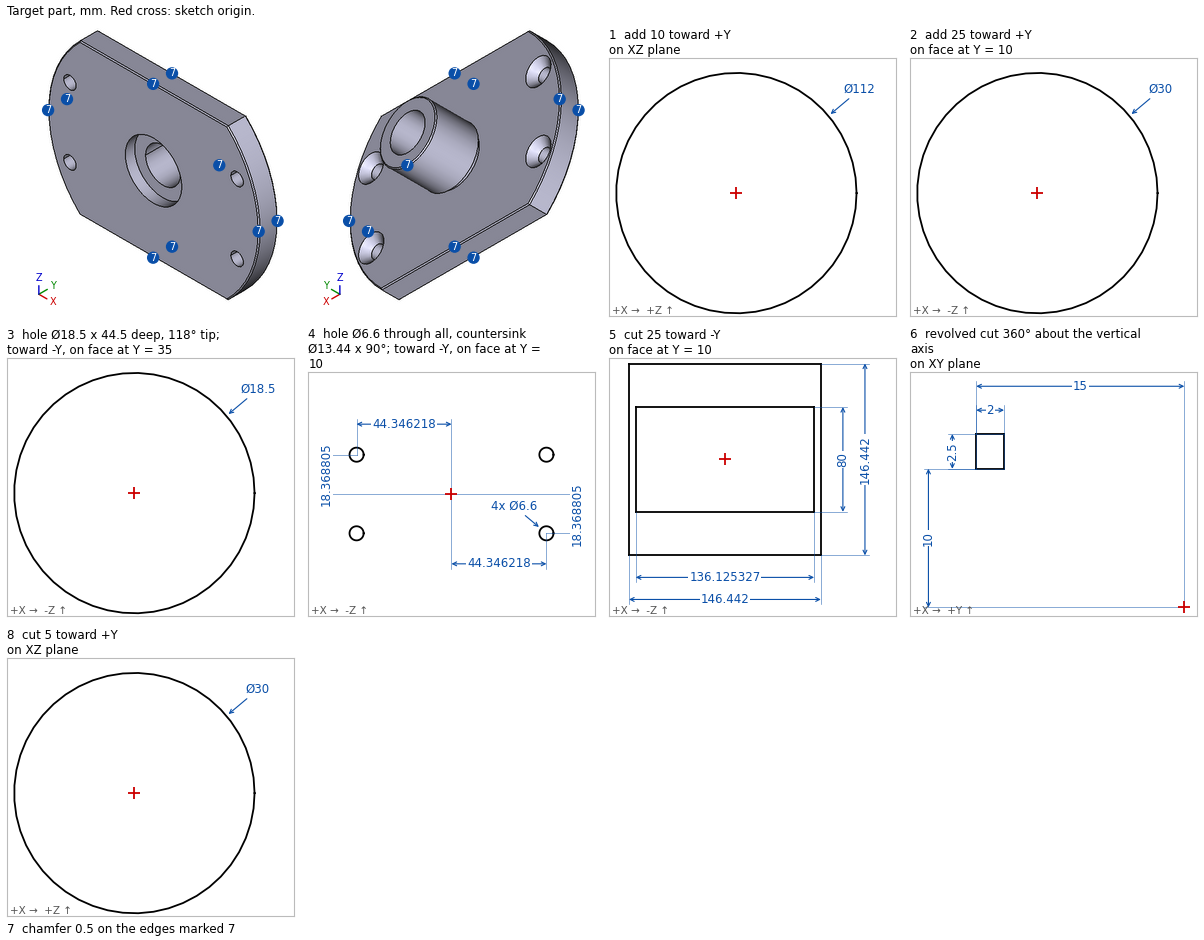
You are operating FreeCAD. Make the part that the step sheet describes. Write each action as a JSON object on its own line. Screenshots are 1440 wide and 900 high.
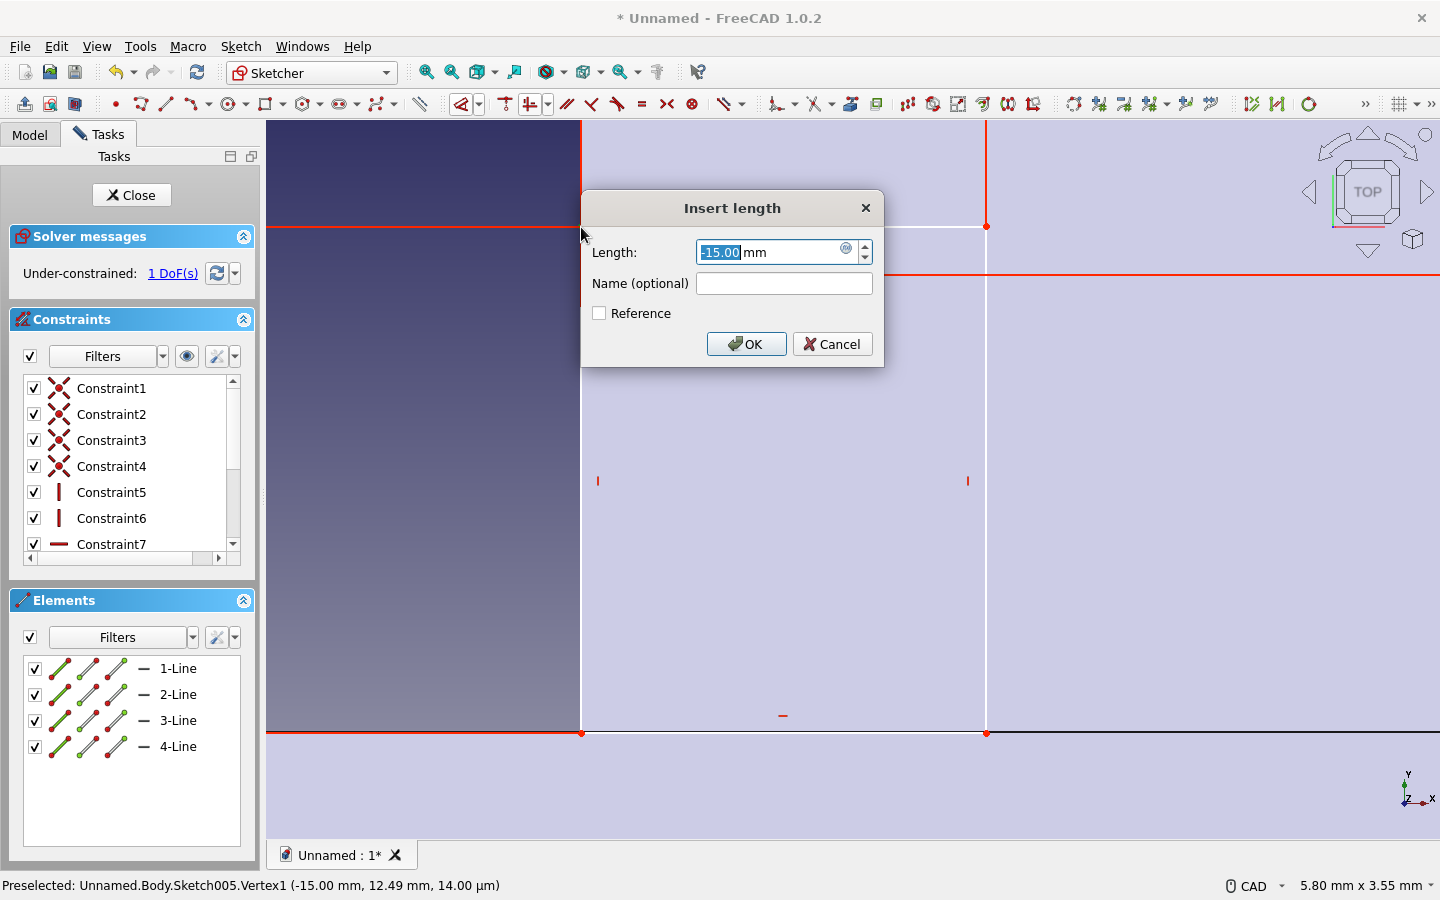
{"action": "type", "text": "-15"}
{"action": "key", "text": "Return"}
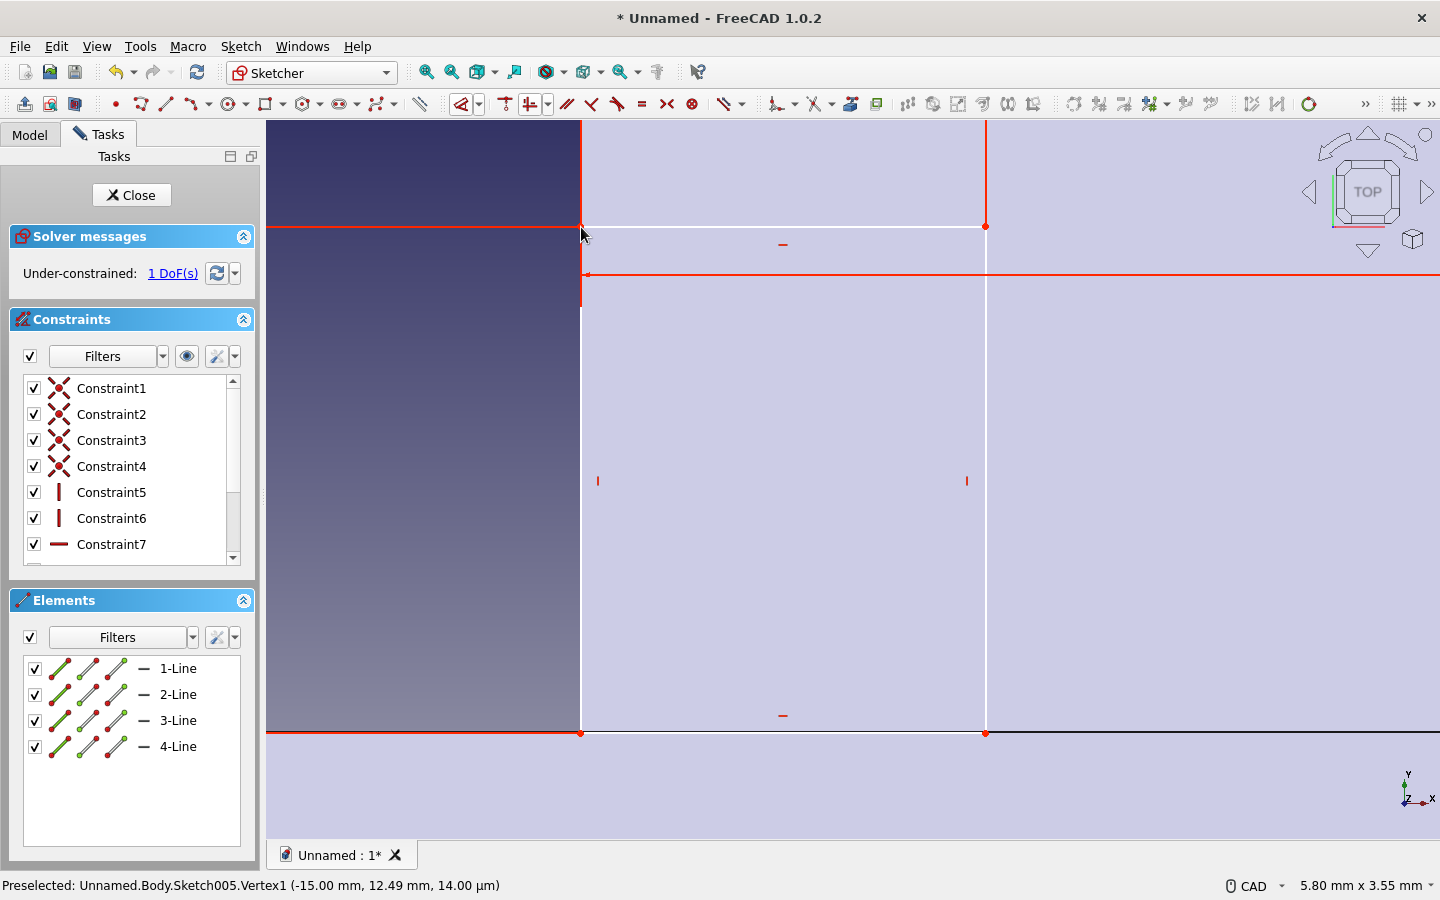
{"action": "left_click", "coordinate": [581, 733]}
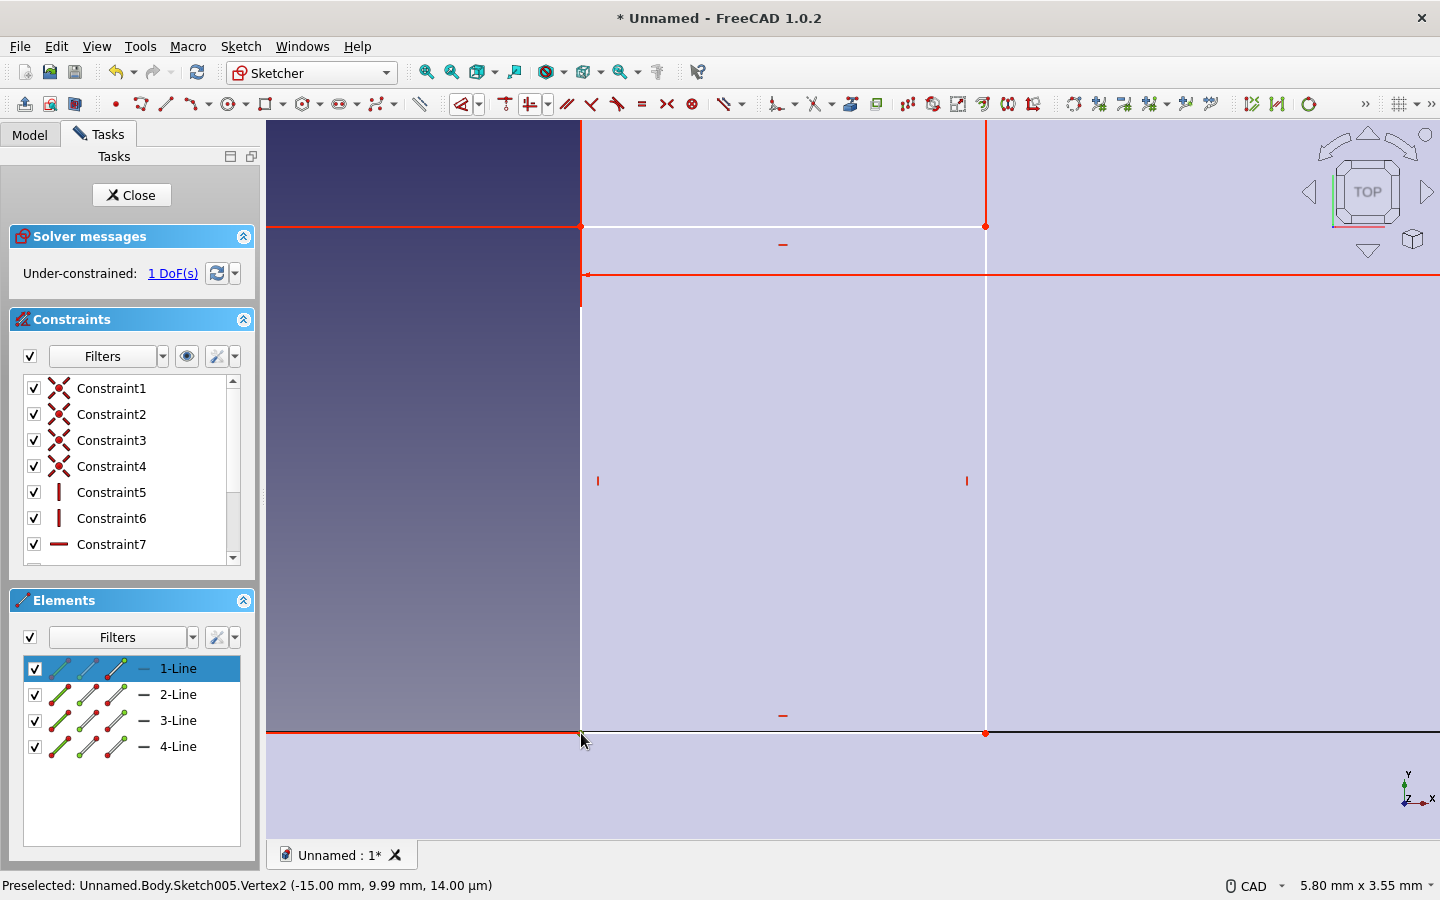
{"action": "key", "text": "i"}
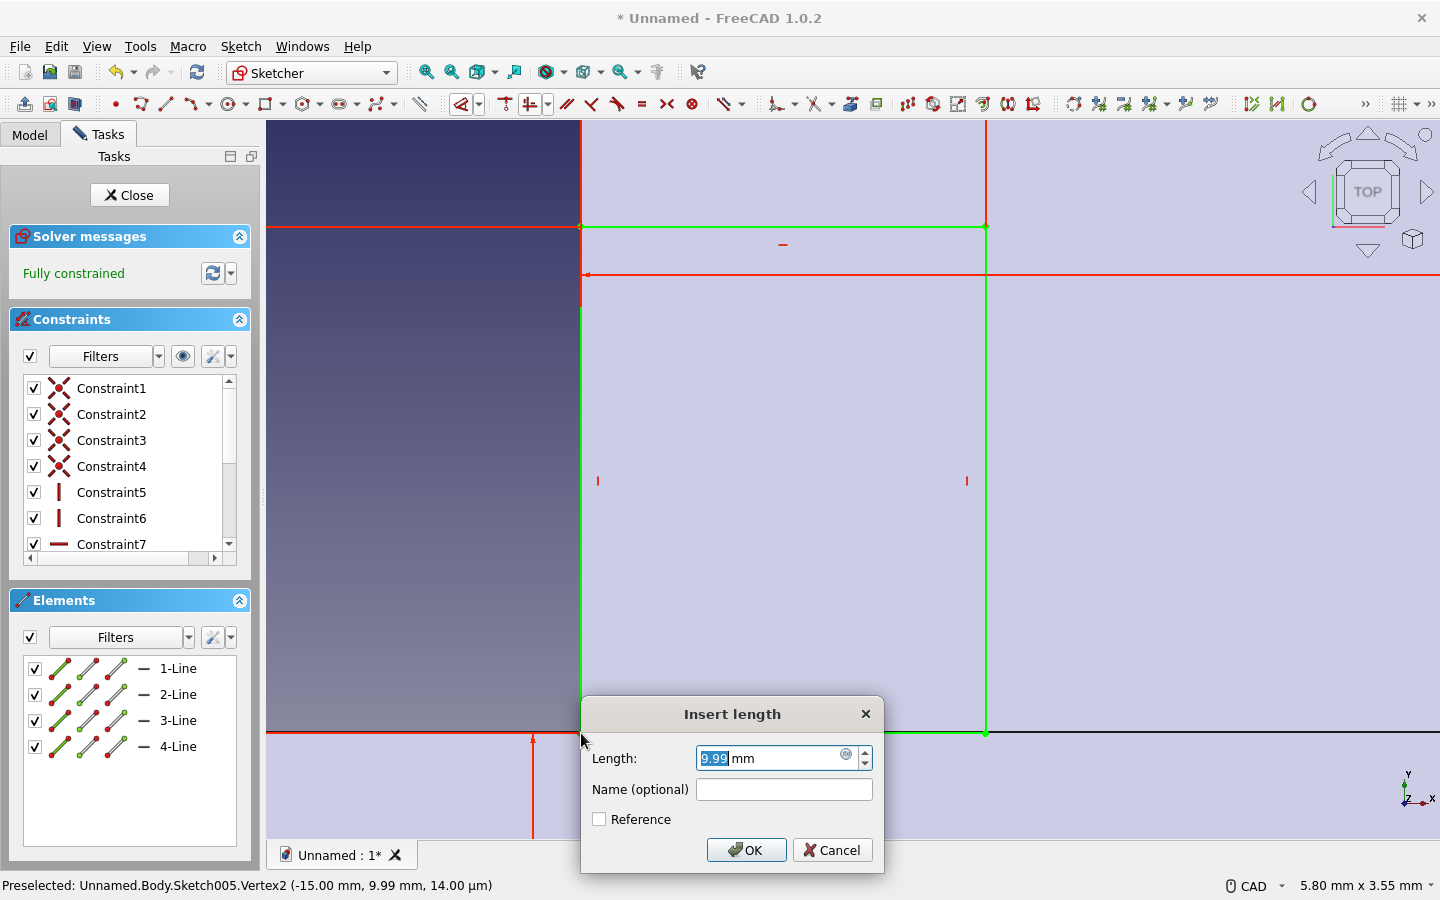
{"action": "type", "text": "10"}
{"action": "key", "text": "Return"}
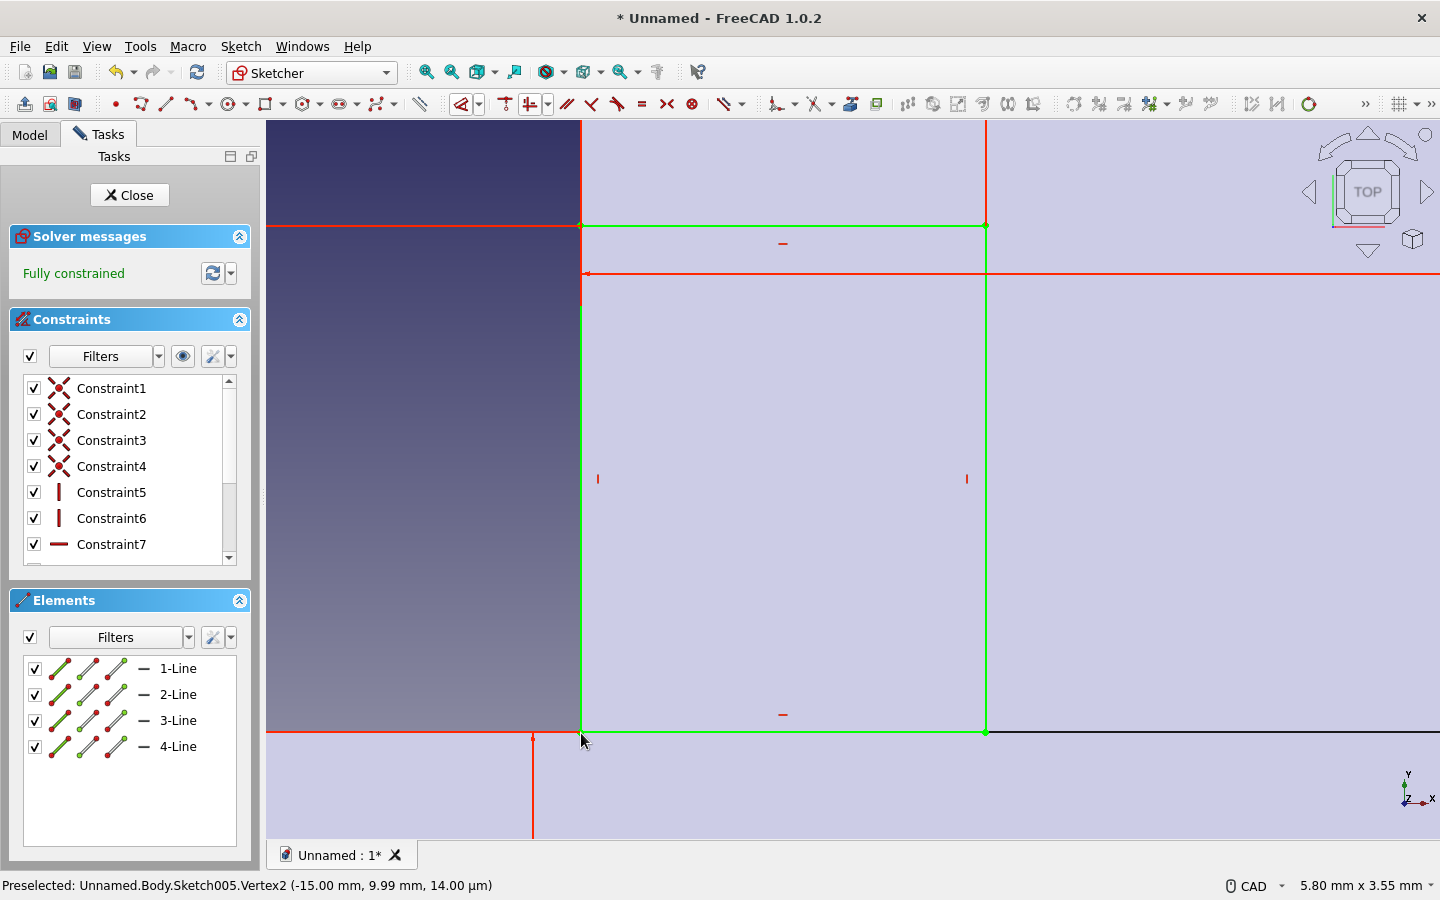
{"action": "left_click", "coordinate": [130, 195]}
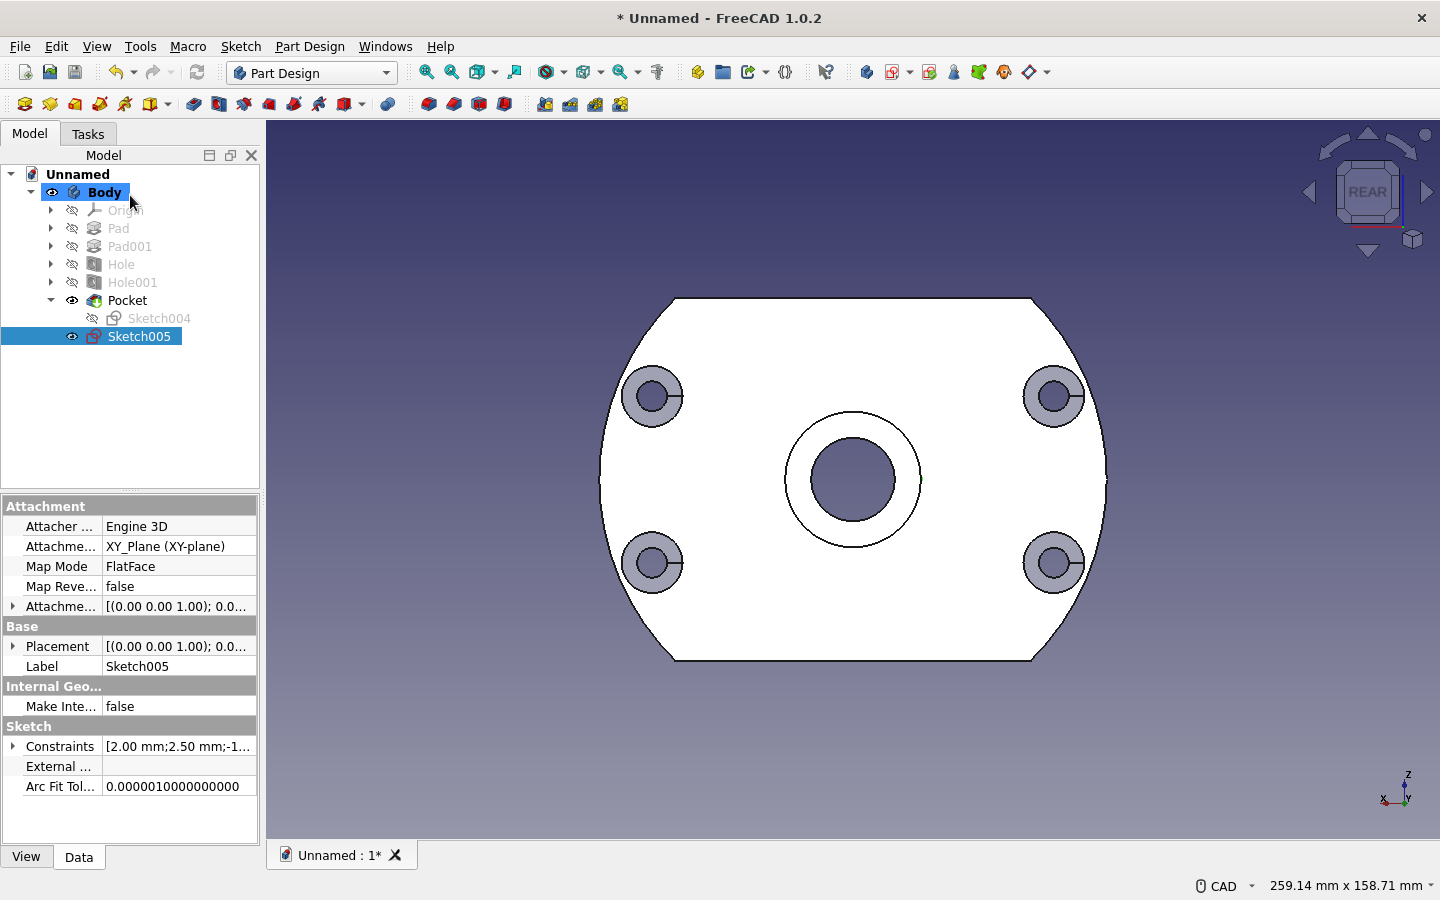
{"action": "left_click", "coordinate": [244, 104]}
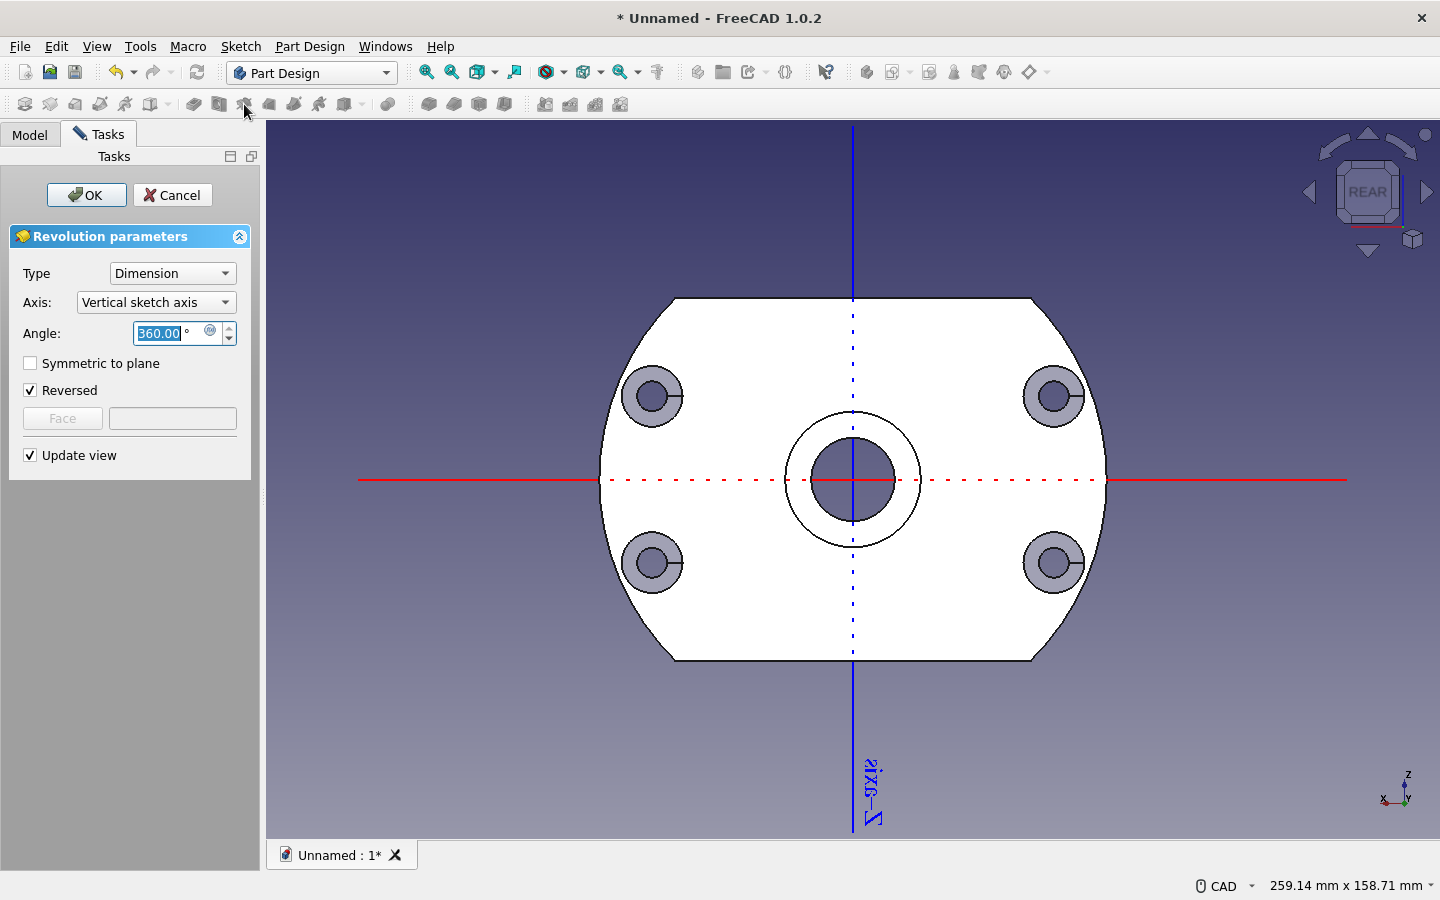
{"action": "left_click", "coordinate": [87, 195]}